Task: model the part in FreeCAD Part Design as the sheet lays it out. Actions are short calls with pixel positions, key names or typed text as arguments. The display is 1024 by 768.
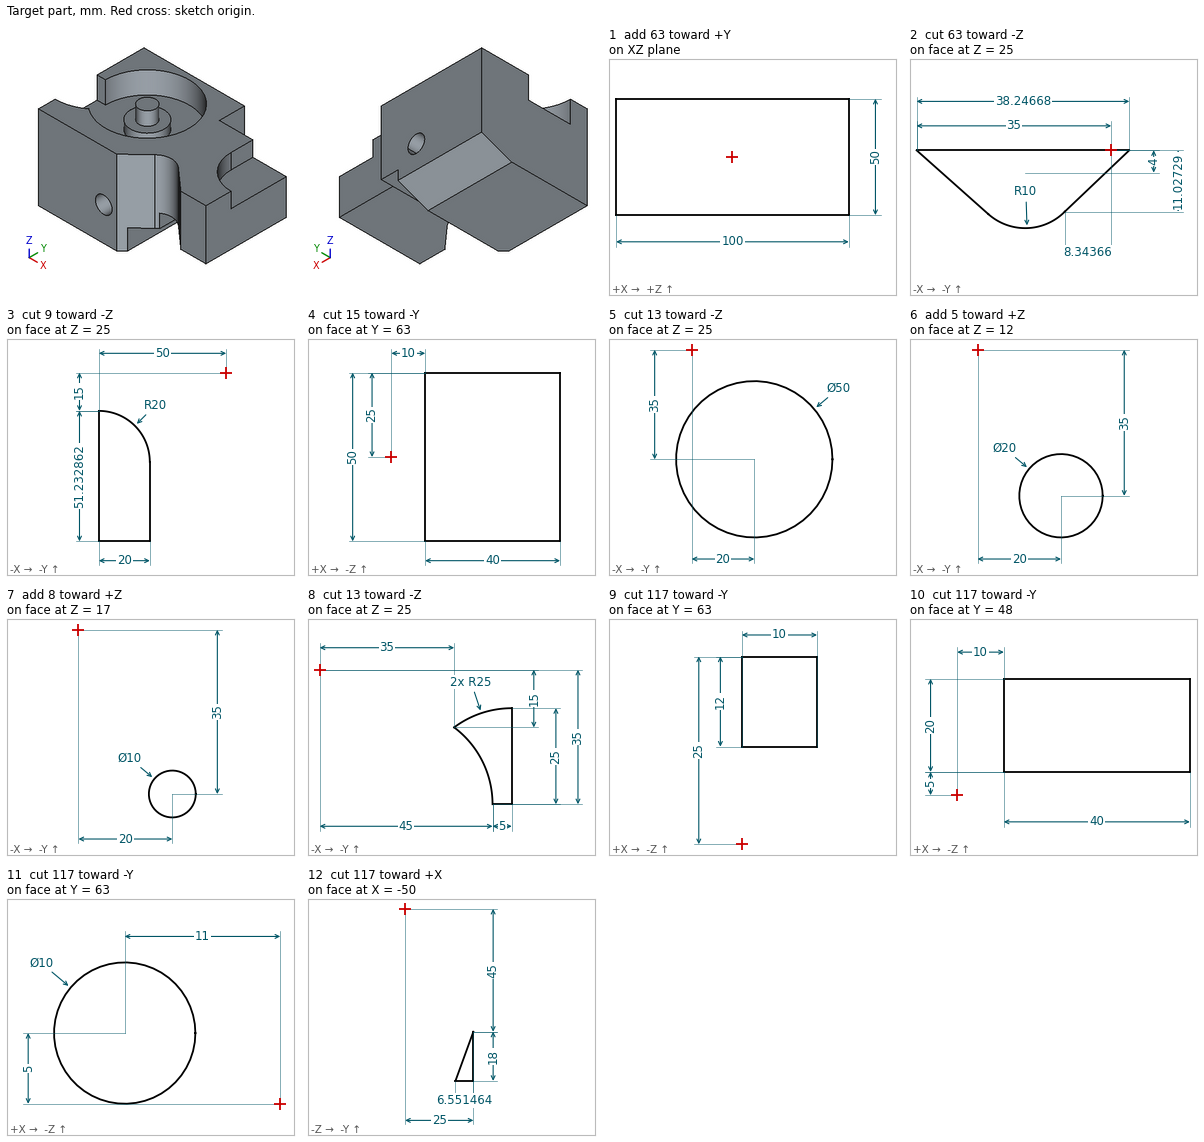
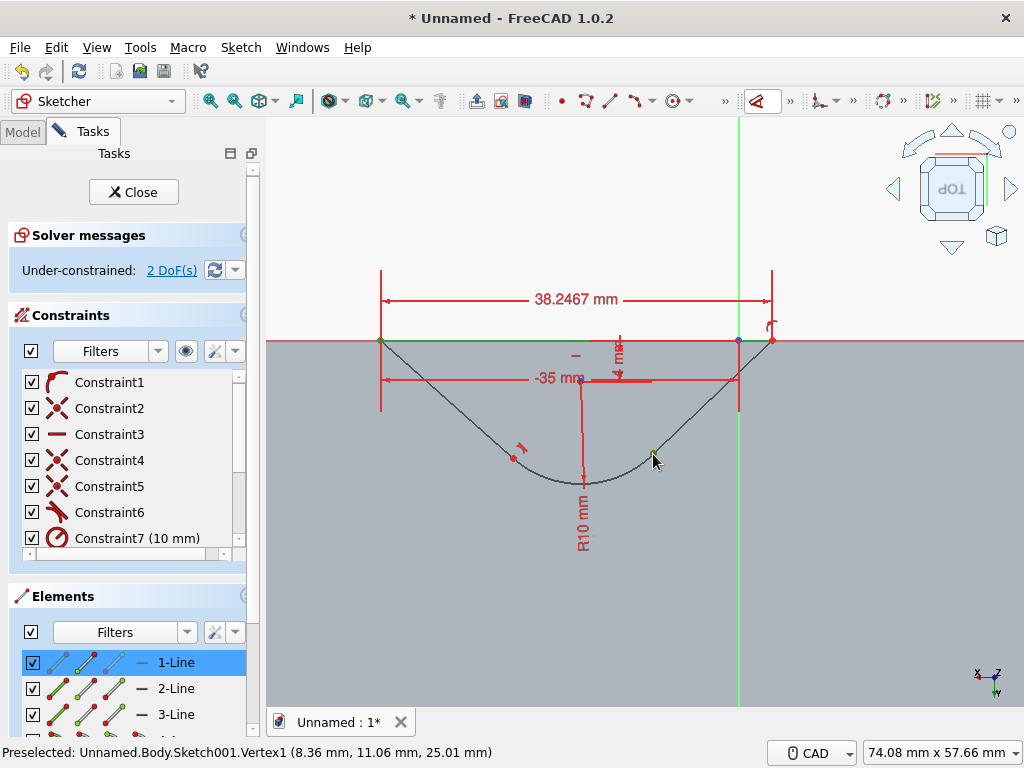
key(l)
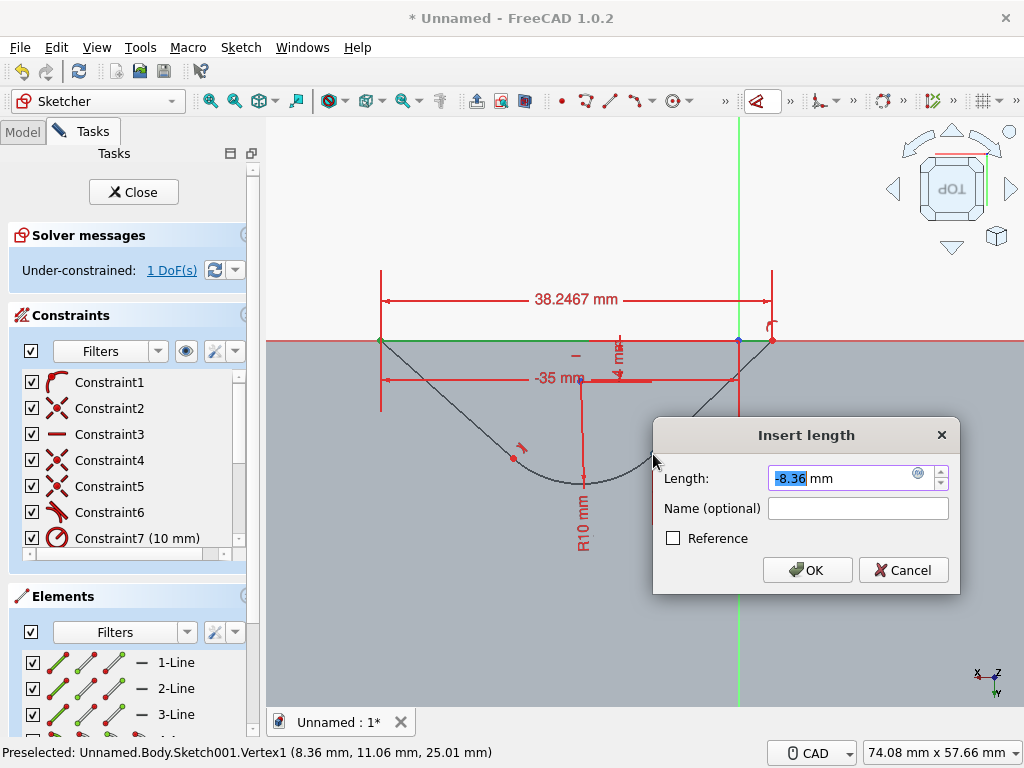
text(-8.34366)
key(Return)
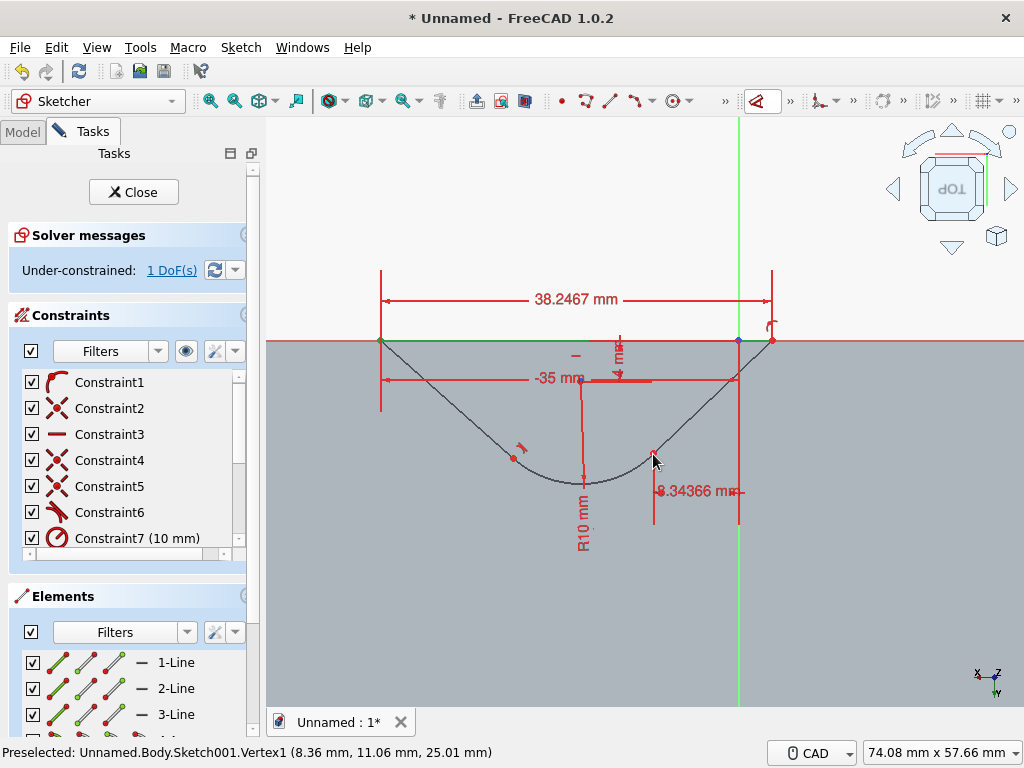
click(654, 454)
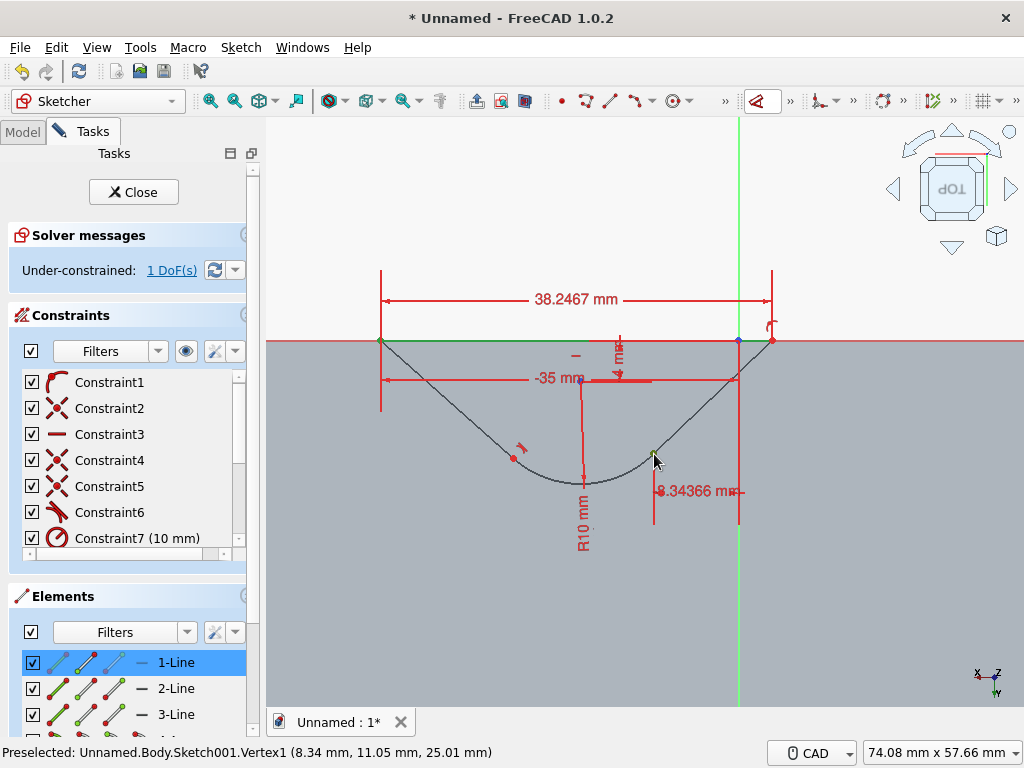
click(776, 102)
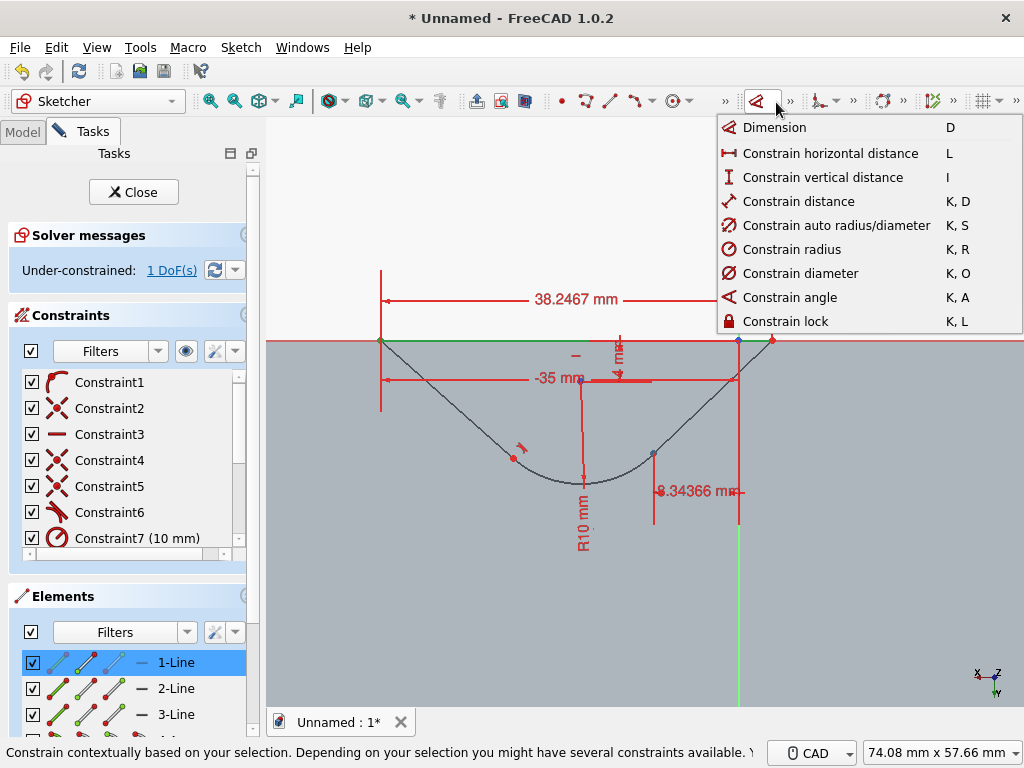
click(870, 177)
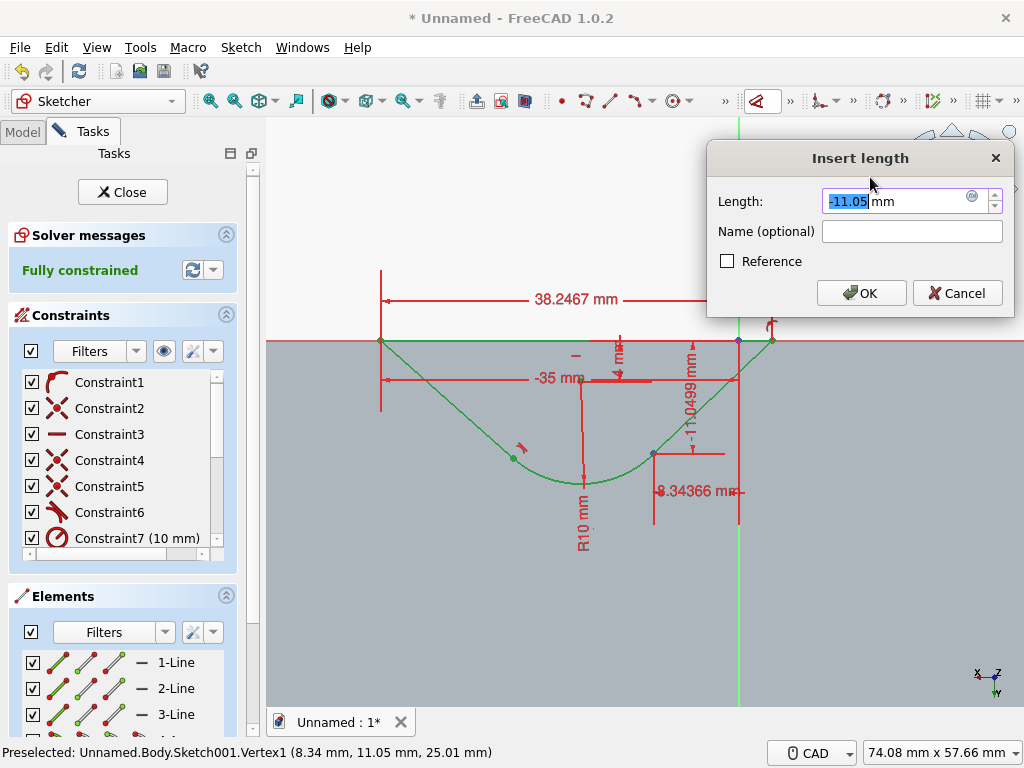
text(-11.02729)
key(Return)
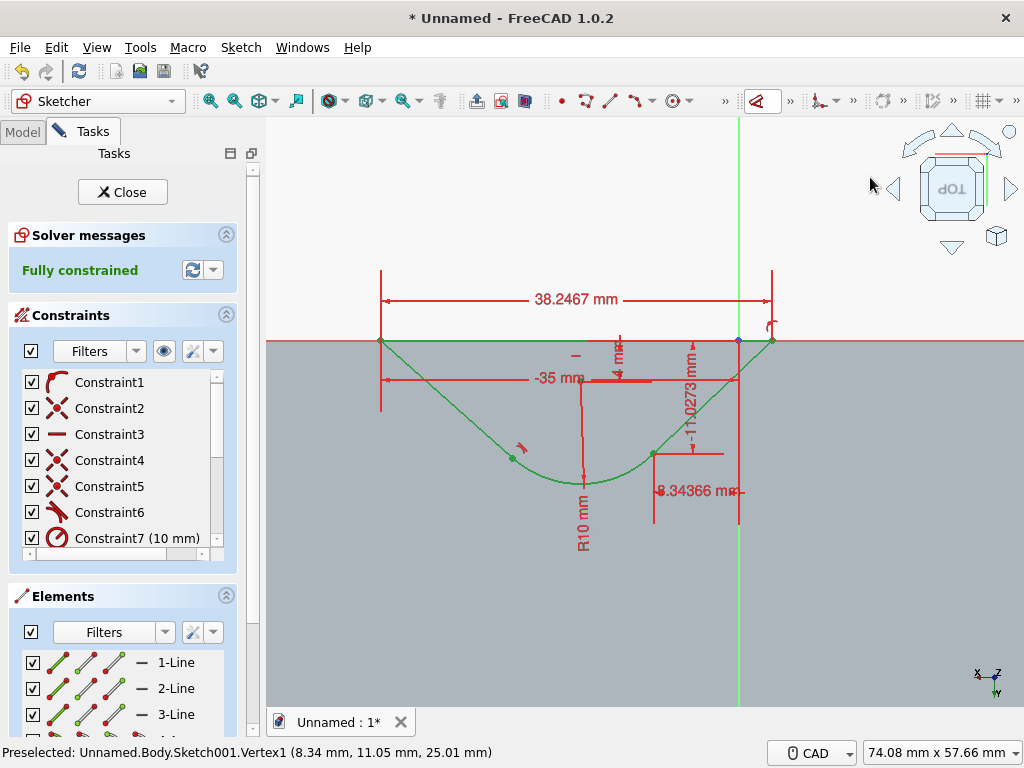
click(123, 192)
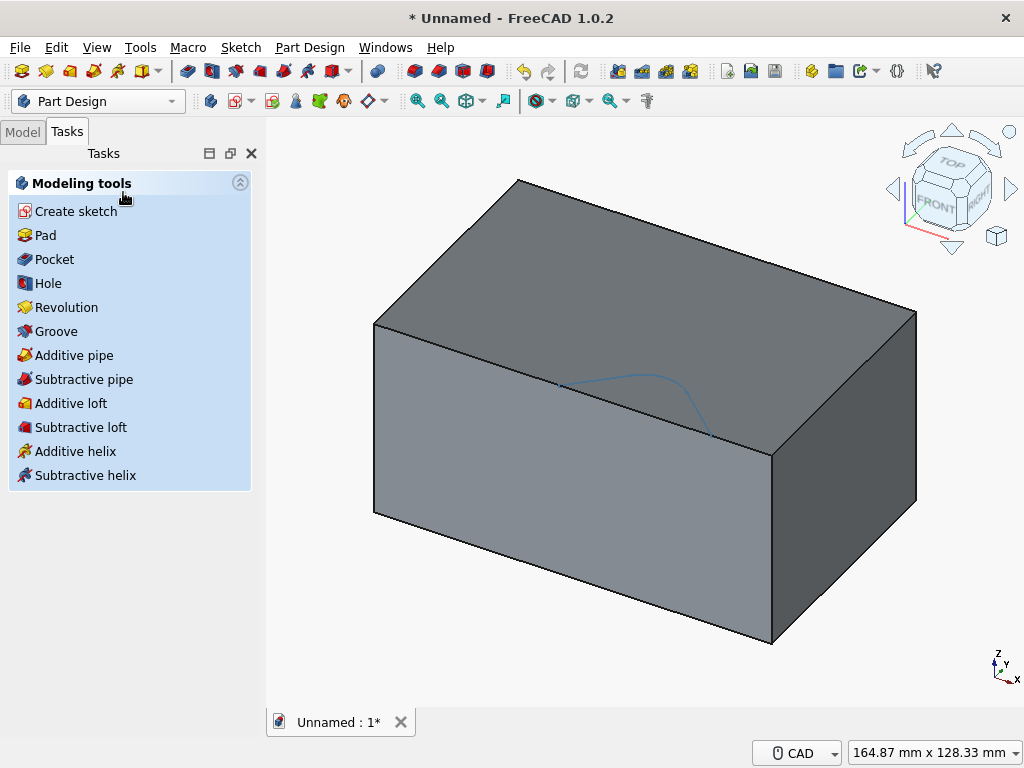
click(188, 72)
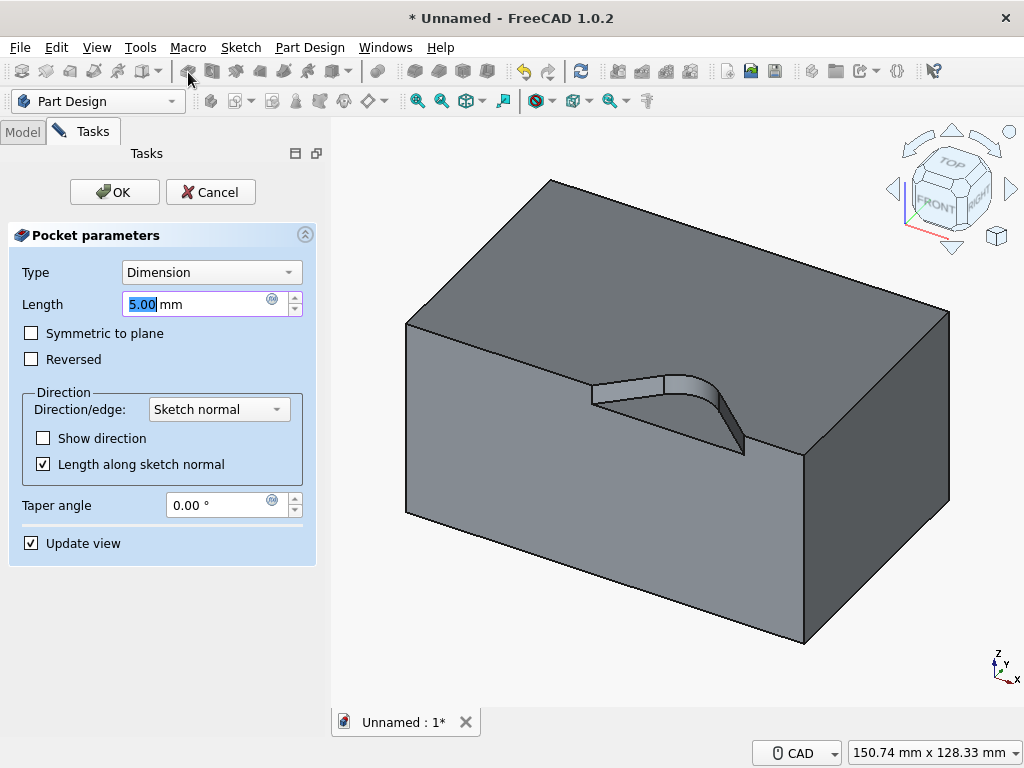
text(63)
key(Tab)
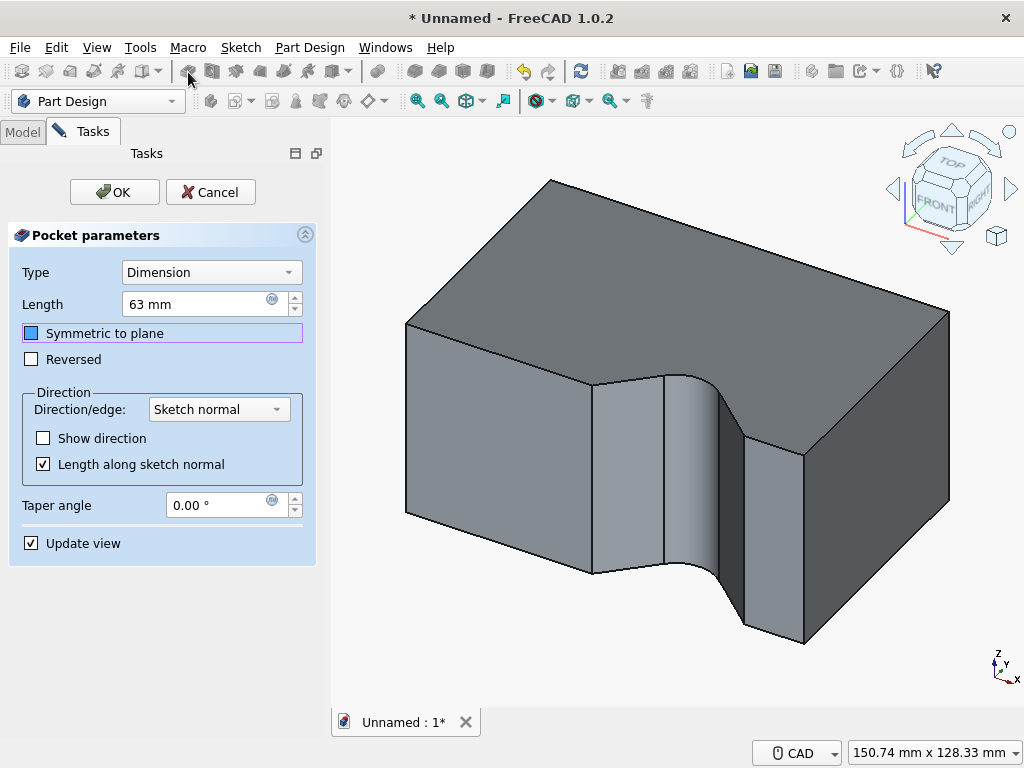
click(115, 192)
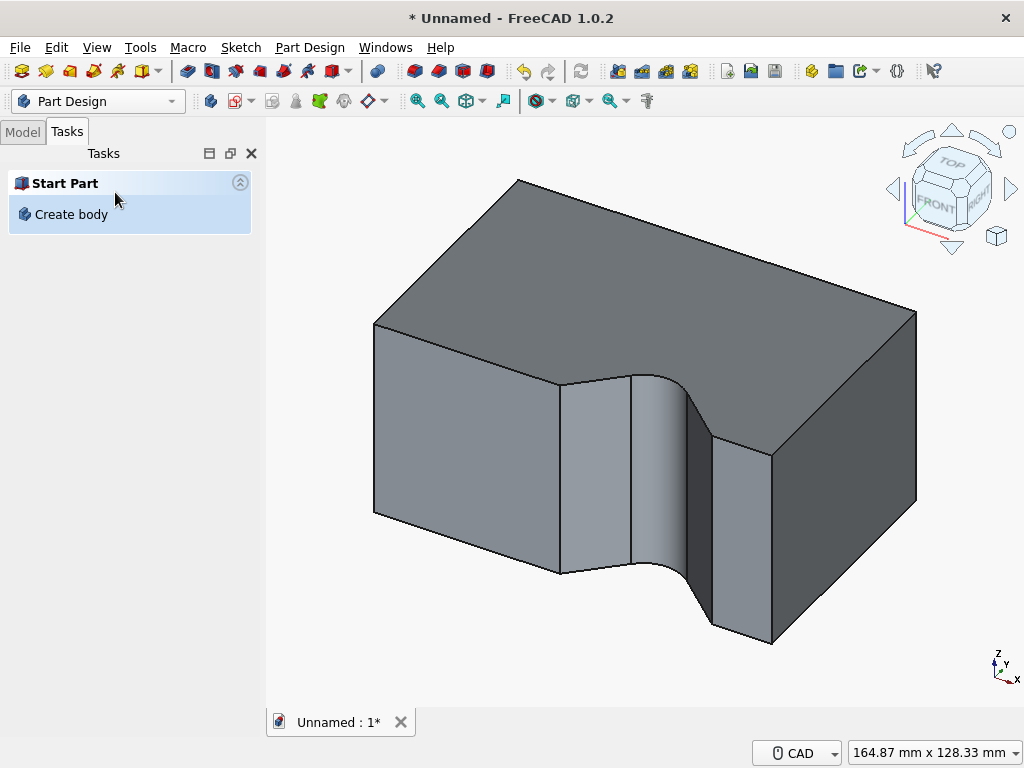
click(588, 298)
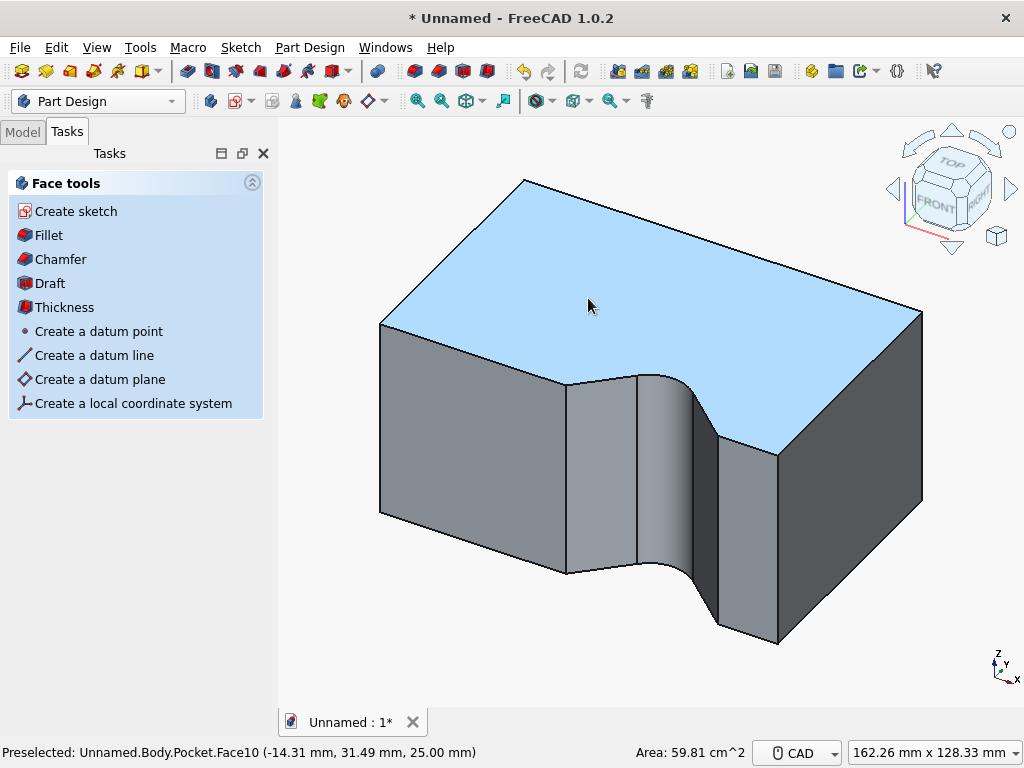
click(236, 102)